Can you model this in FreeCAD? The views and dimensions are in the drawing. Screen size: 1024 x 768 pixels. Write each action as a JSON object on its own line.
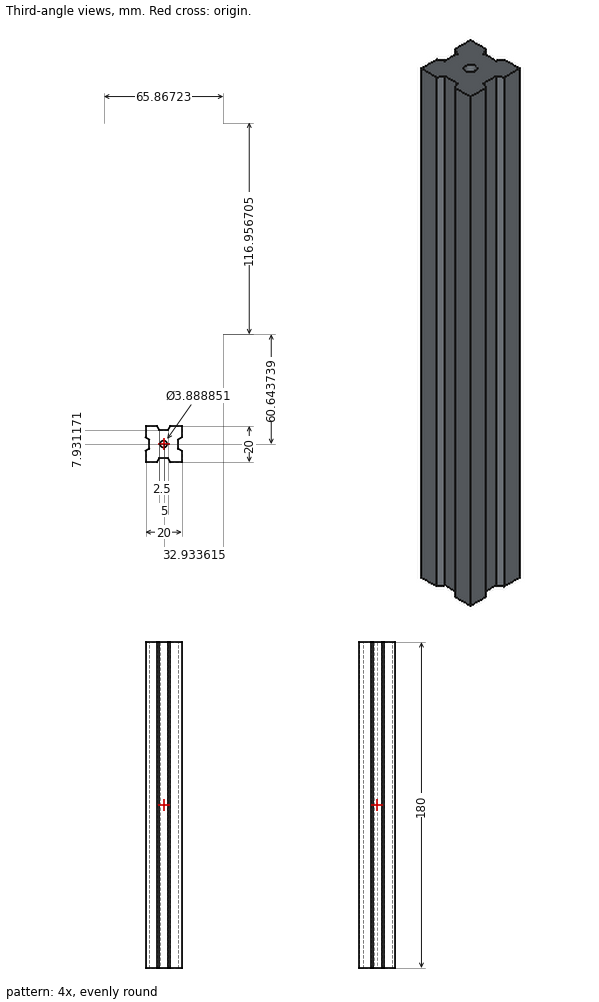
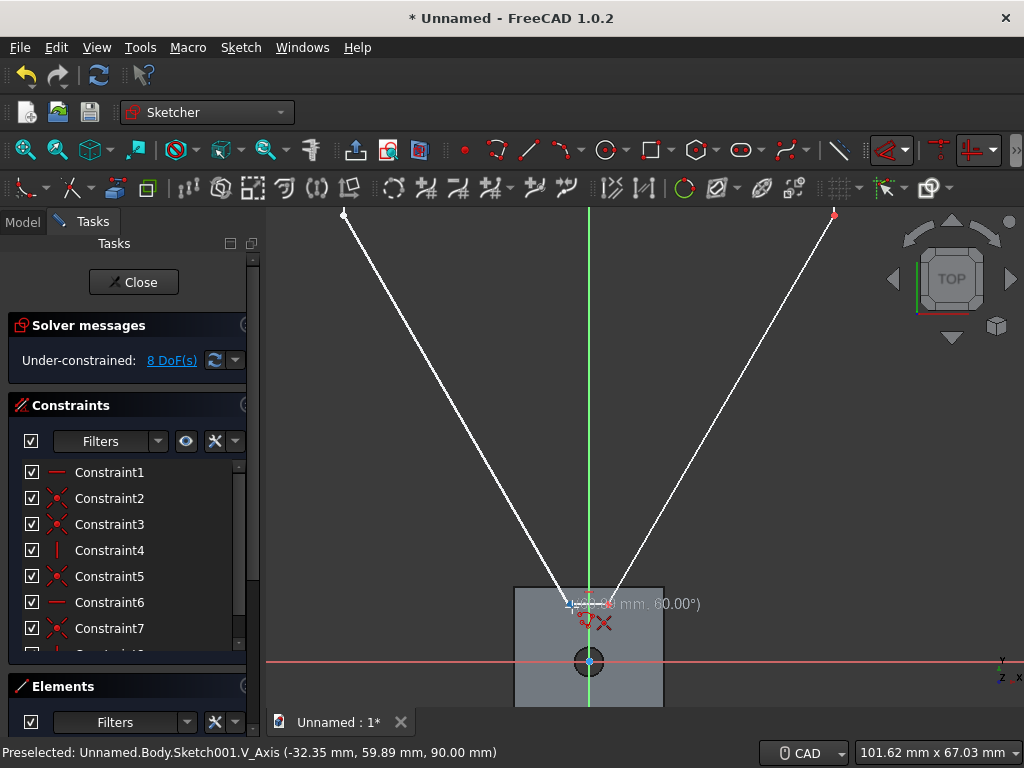
{"action": "left_click", "coordinate": [570, 604]}
{"action": "key", "text": "Escape"}
{"action": "key", "text": "Escape"}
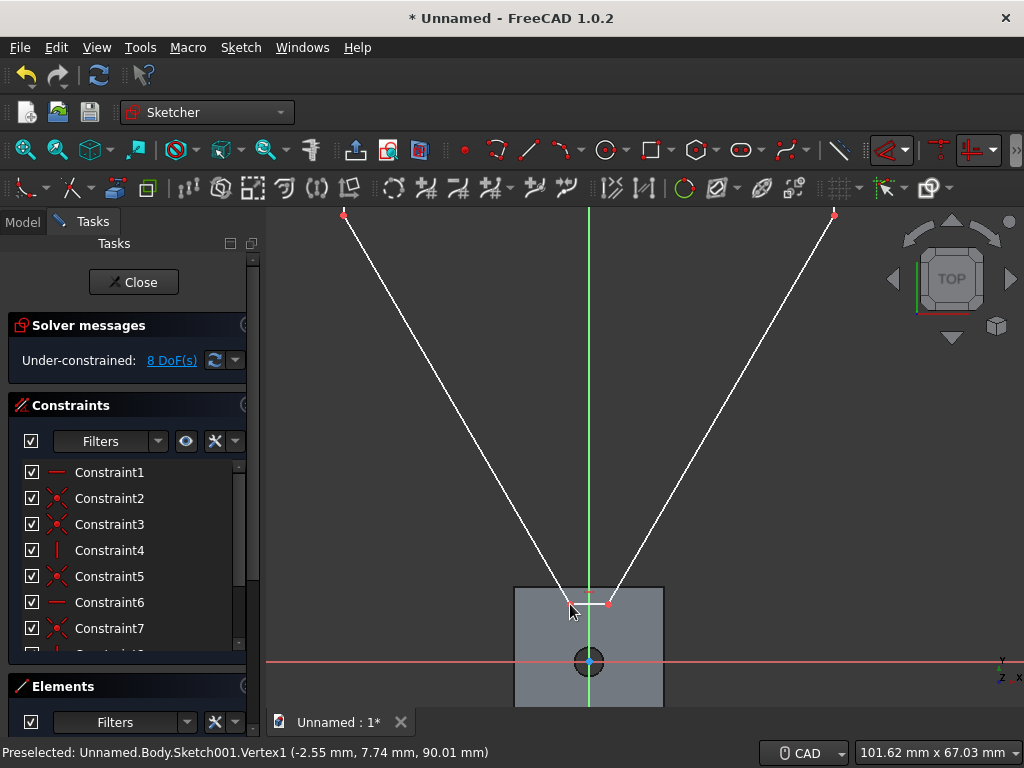
{"action": "left_click", "coordinate": [886, 150]}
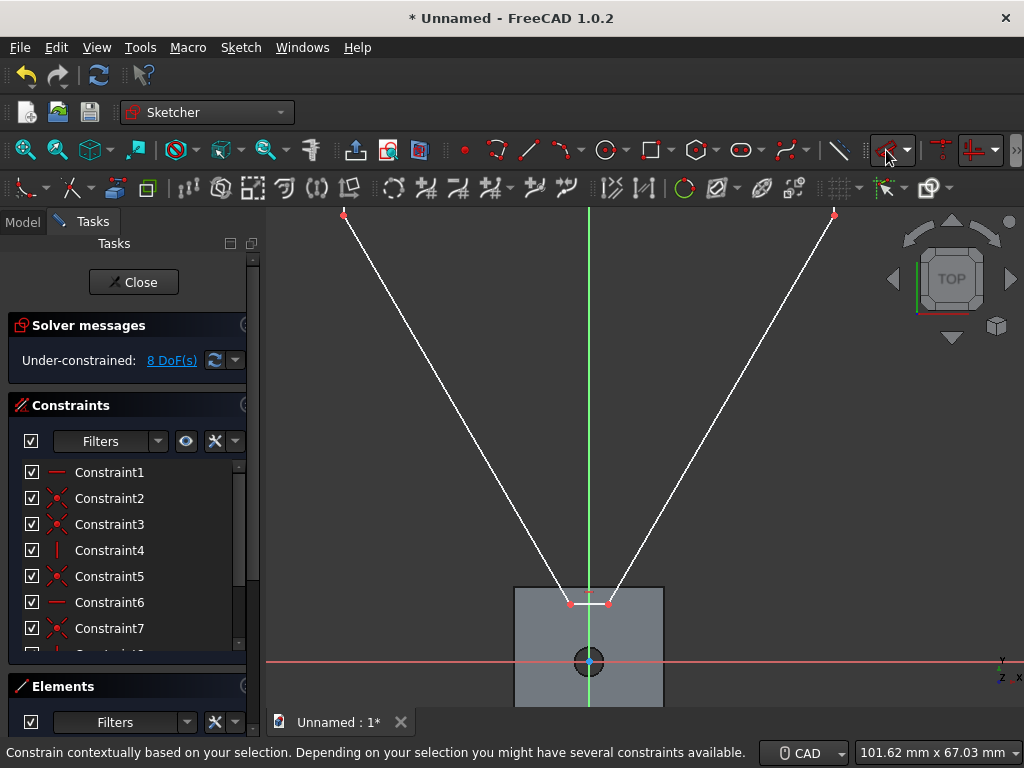
{"action": "left_click", "coordinate": [585, 604]}
{"action": "left_click", "coordinate": [576, 638]}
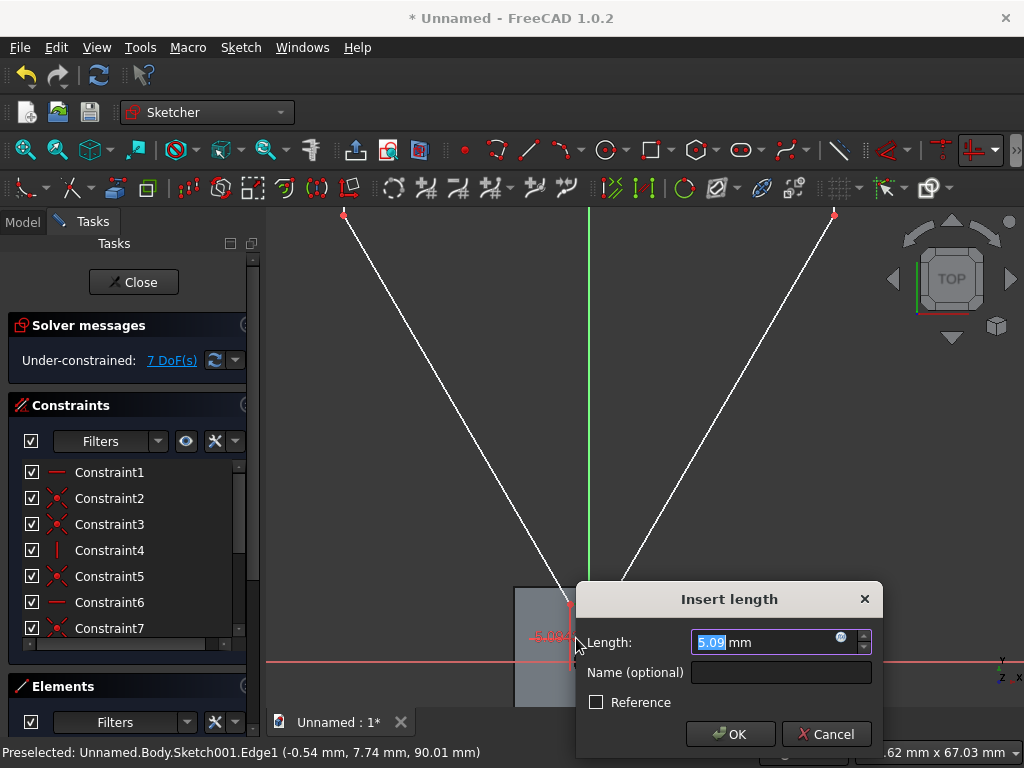
{"action": "type", "text": "5"}
{"action": "key", "text": "Return"}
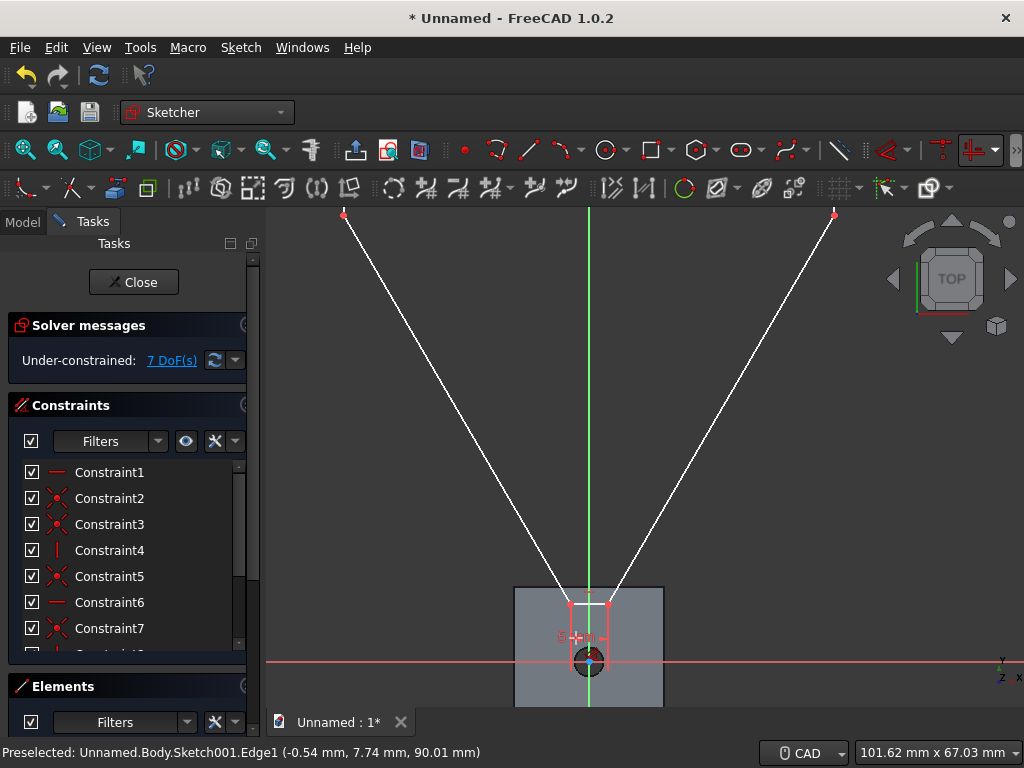
{"action": "scroll", "coordinate": [571, 604], "scroll_direction": "up", "scroll_amount": 4}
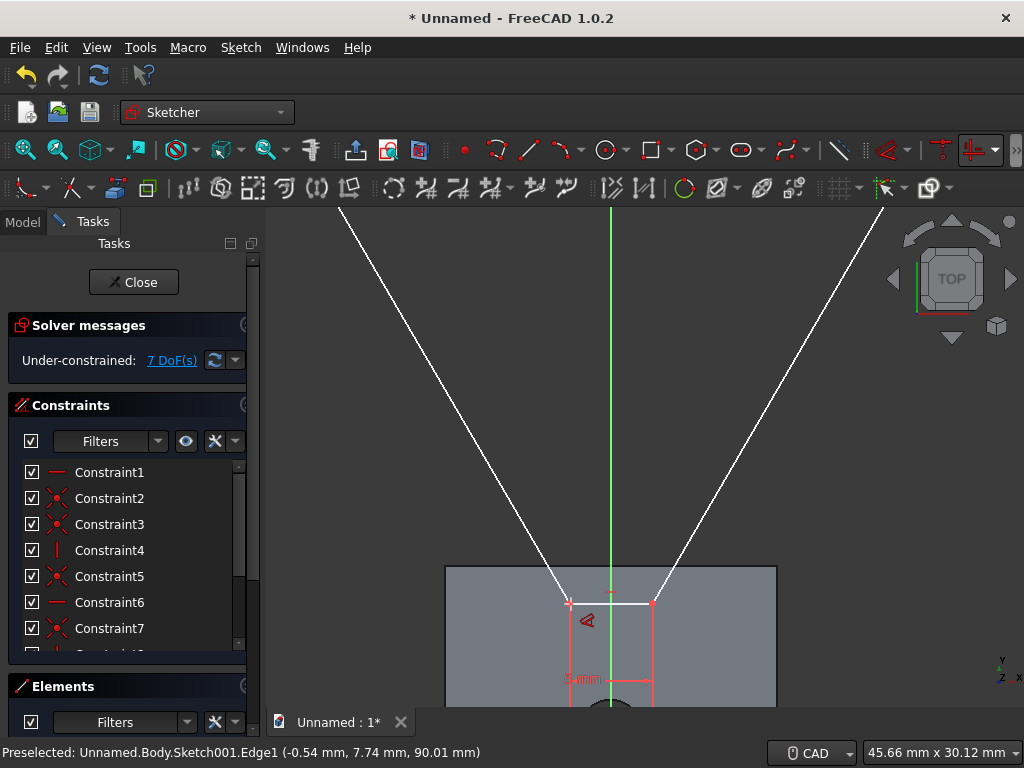
{"action": "left_click", "coordinate": [570, 604]}
{"action": "left_click", "coordinate": [590, 570]}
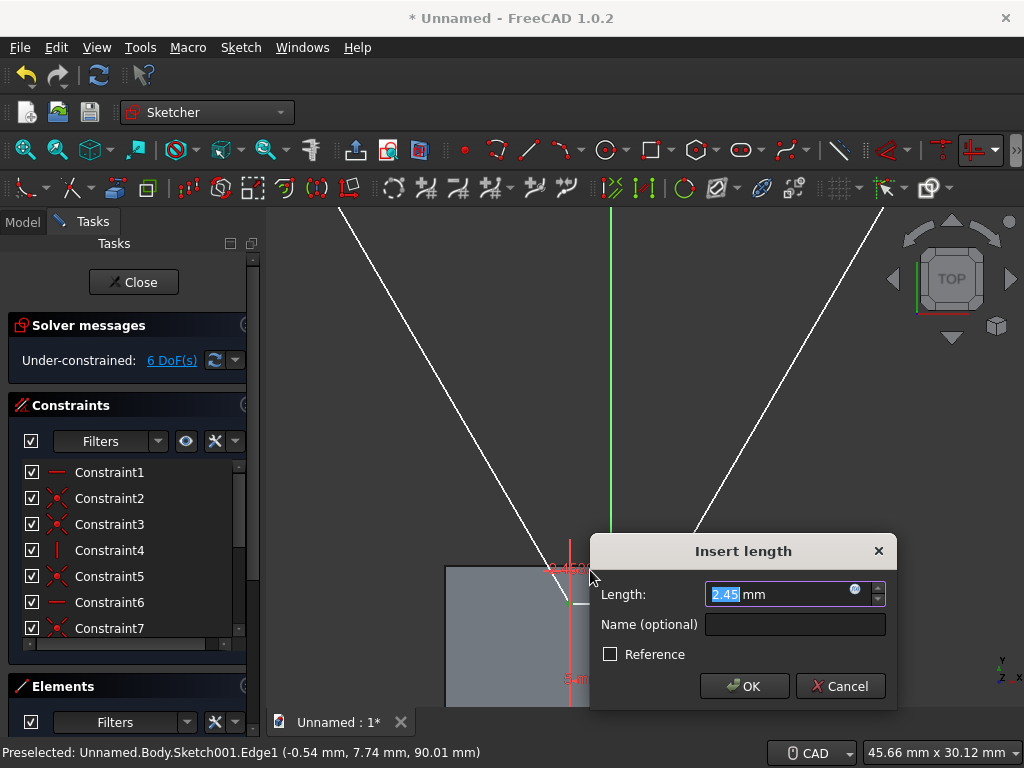
{"action": "type", "text": "2.5"}
{"action": "key", "text": "Return"}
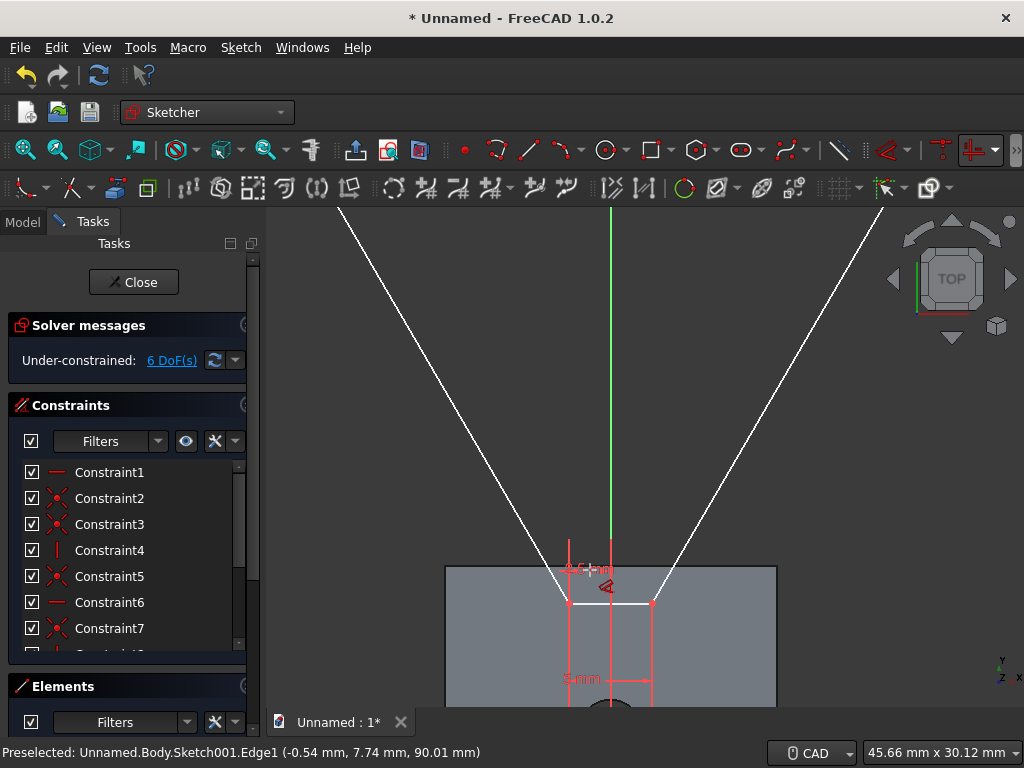
{"action": "scroll", "coordinate": [572, 606], "scroll_direction": "down", "scroll_amount": 11}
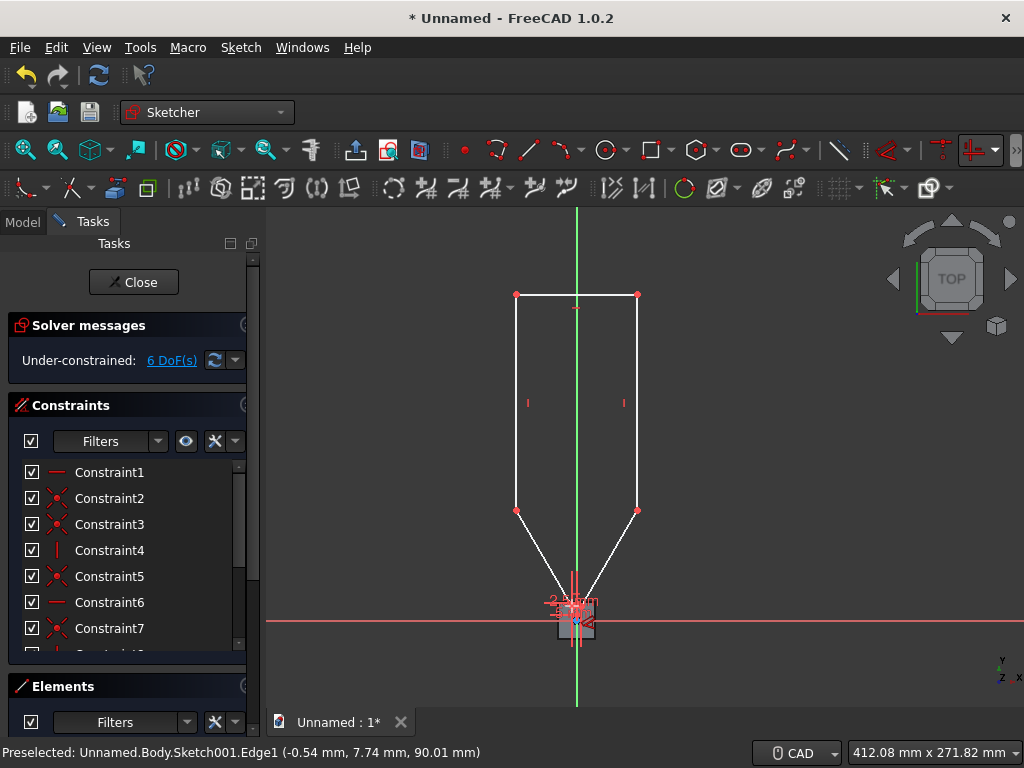
{"action": "left_click", "coordinate": [601, 295]}
{"action": "left_click", "coordinate": [549, 261]}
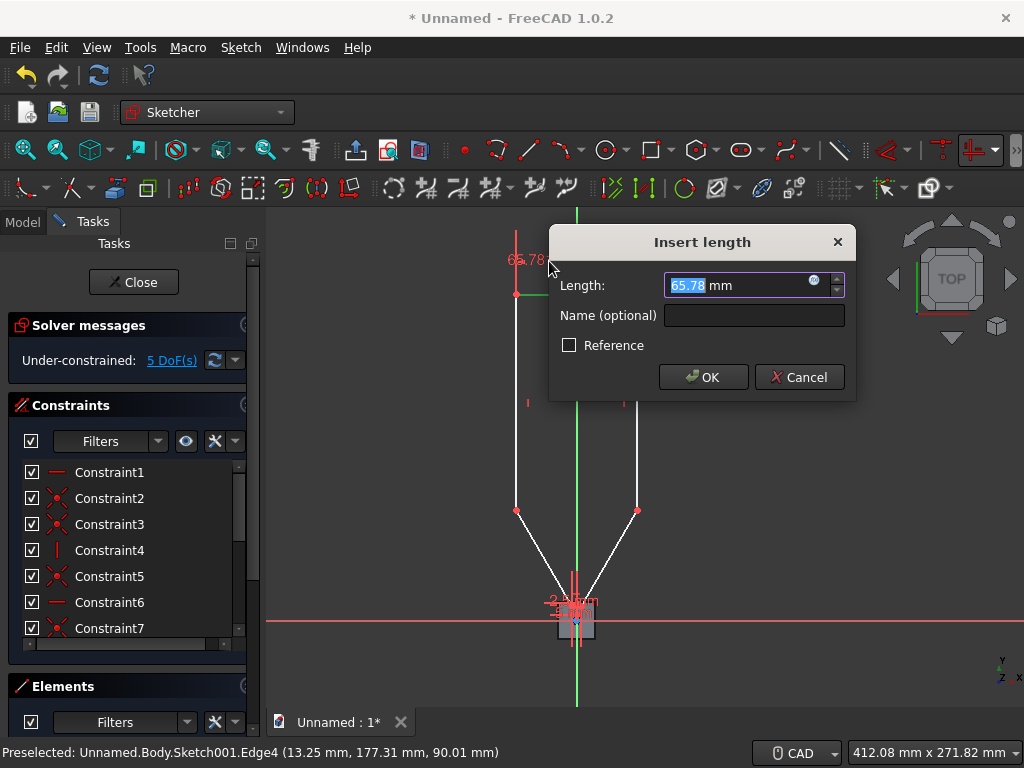
{"action": "type", "text": "65.86723"}
{"action": "key", "text": "Return"}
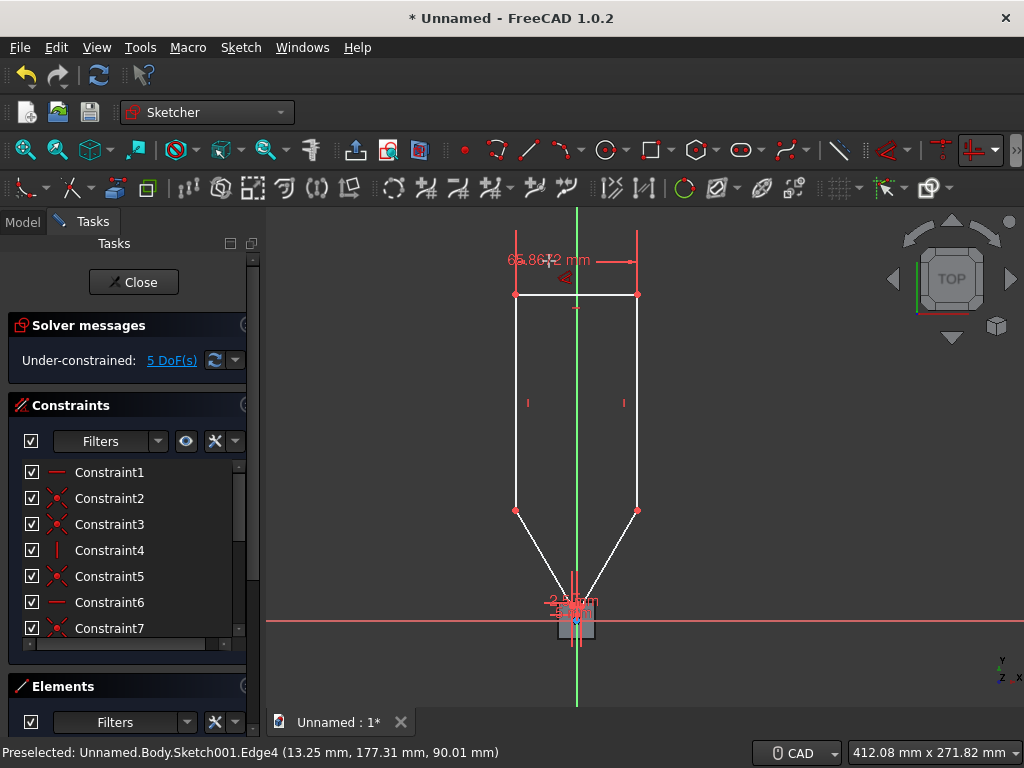
{"action": "scroll", "coordinate": [572, 606], "scroll_direction": "up", "scroll_amount": 6}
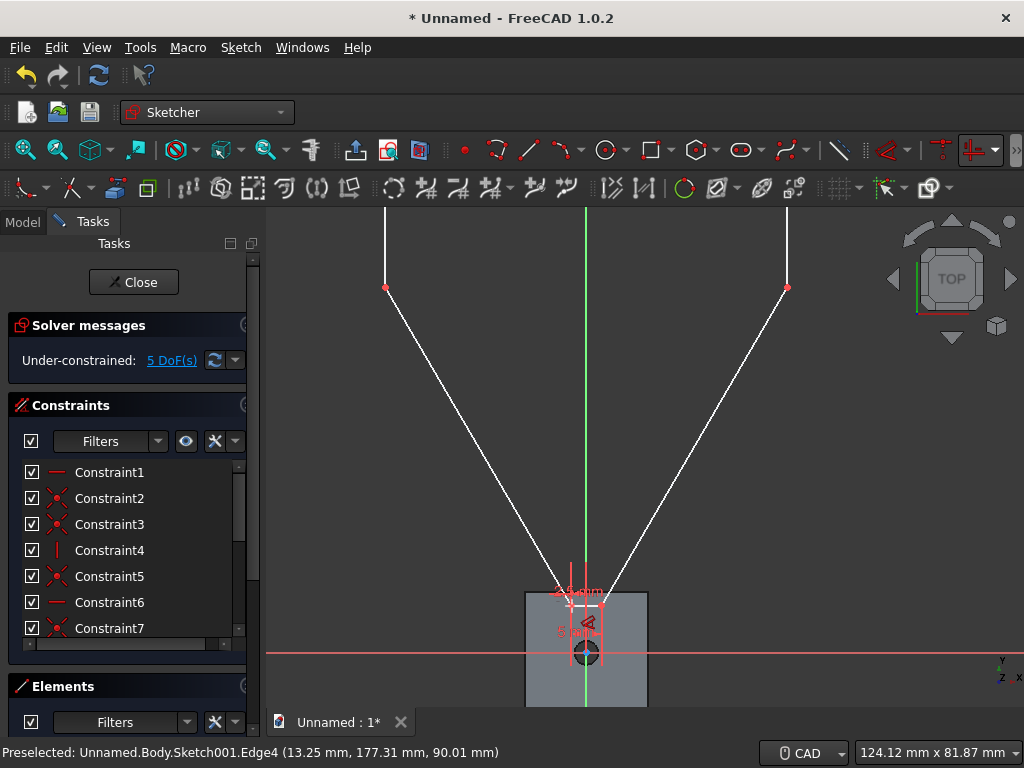
{"action": "left_click", "coordinate": [571, 606]}
{"action": "left_click", "coordinate": [489, 629]}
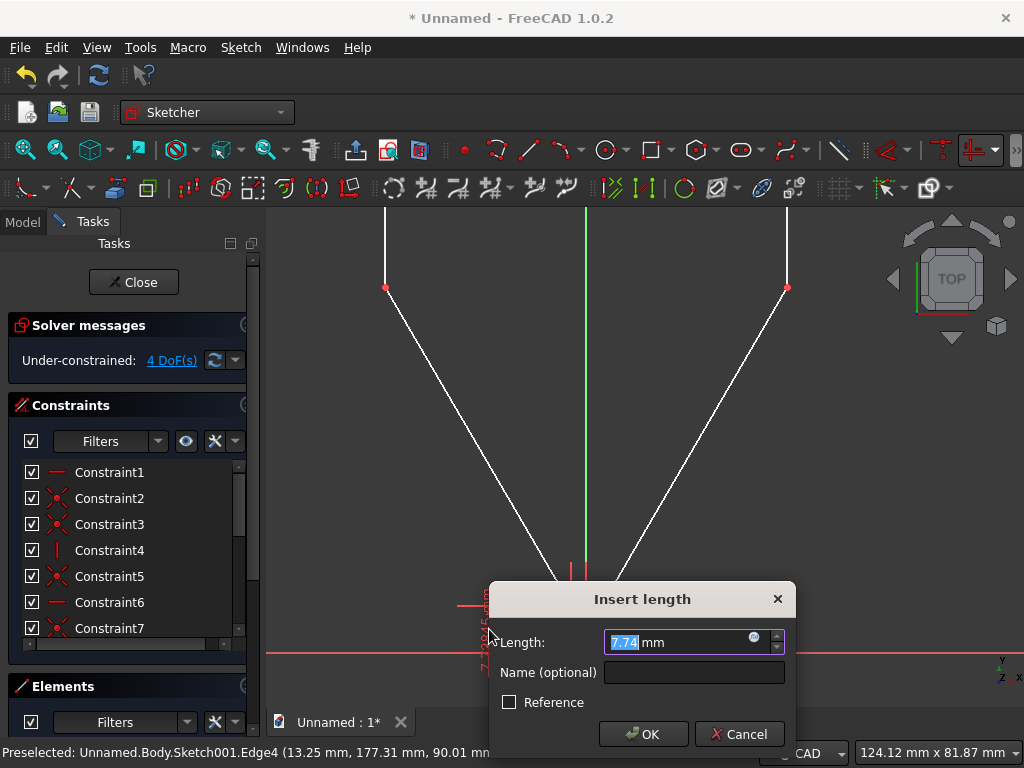
{"action": "type", "text": "7.931171"}
{"action": "key", "text": "Return"}